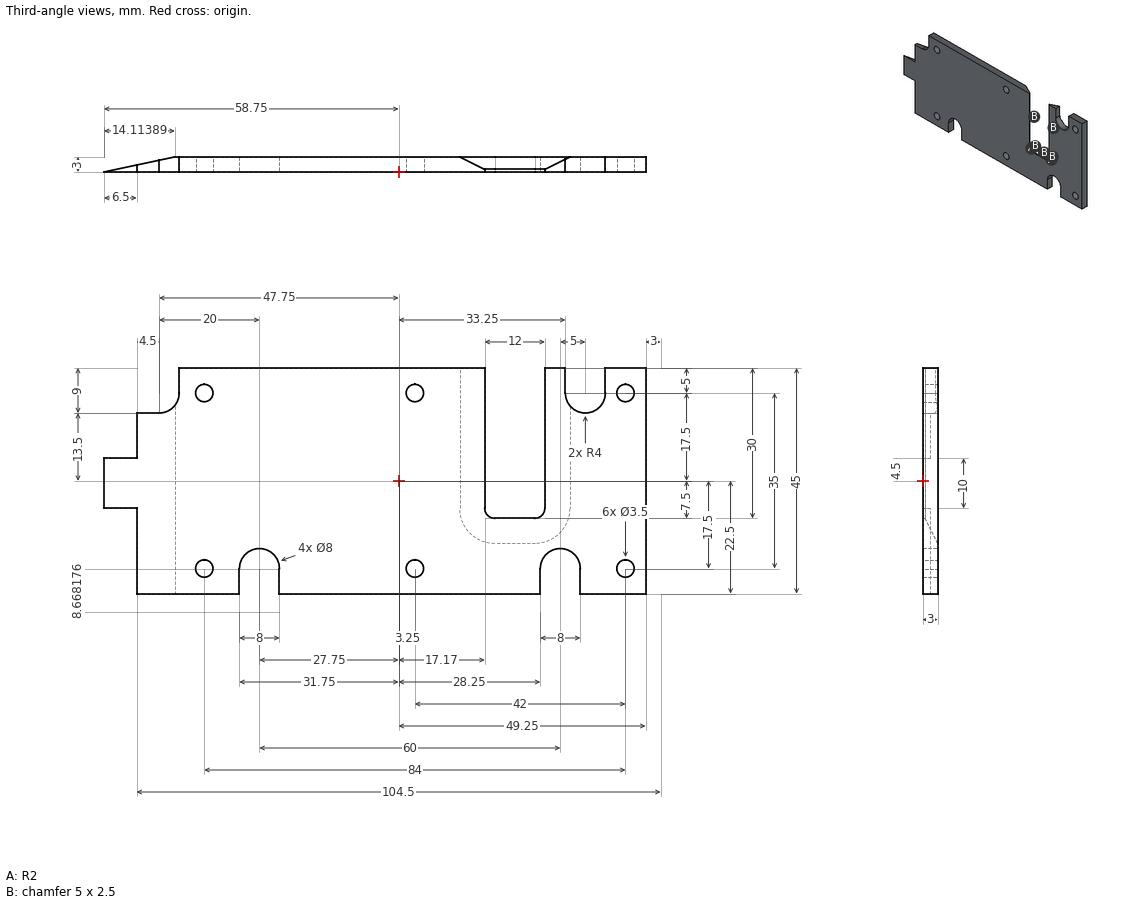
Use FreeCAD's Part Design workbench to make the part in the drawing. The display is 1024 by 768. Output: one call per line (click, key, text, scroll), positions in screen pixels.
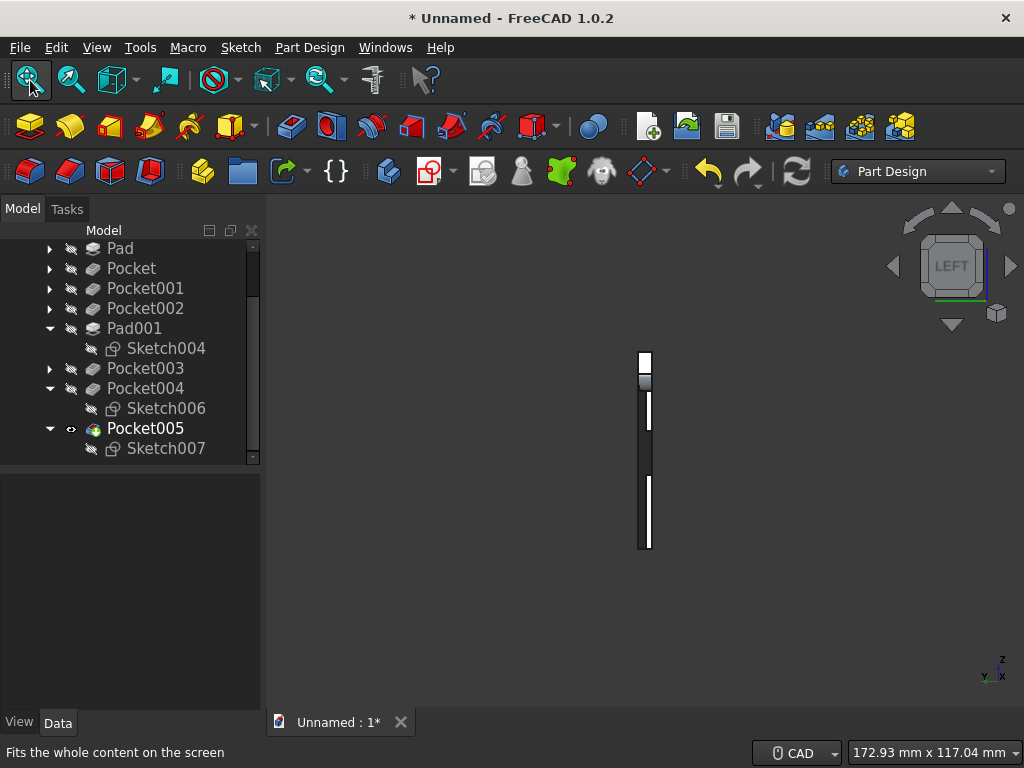
scroll(645, 482, up, 6)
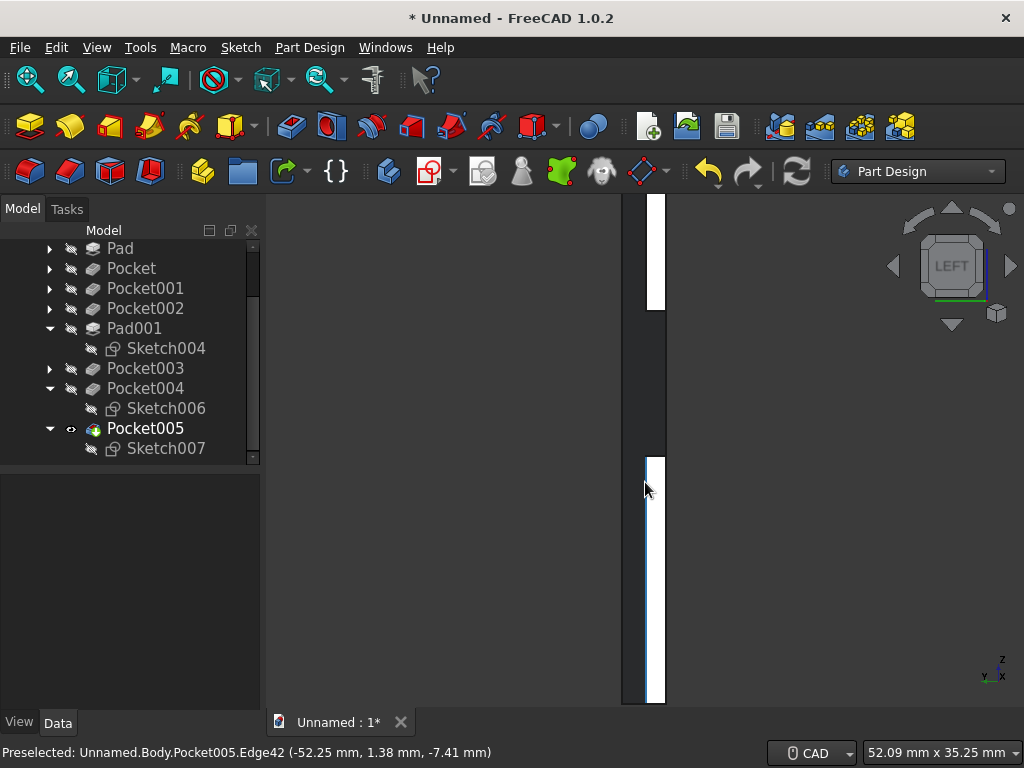
click(32, 80)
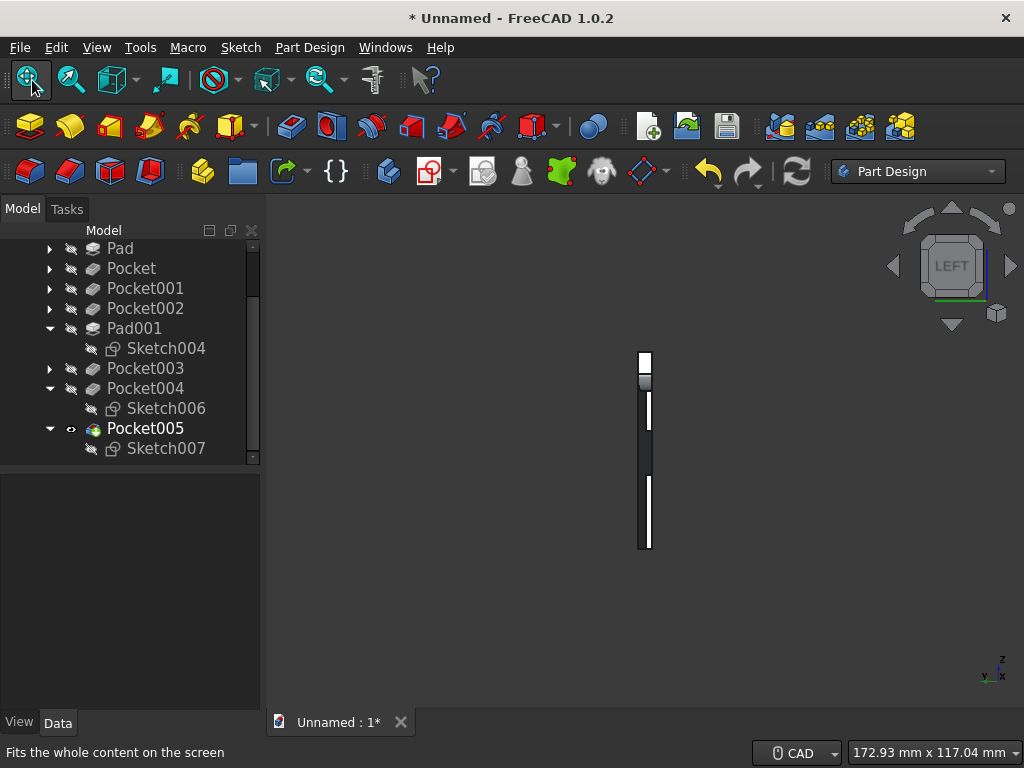
key(v)
key(3)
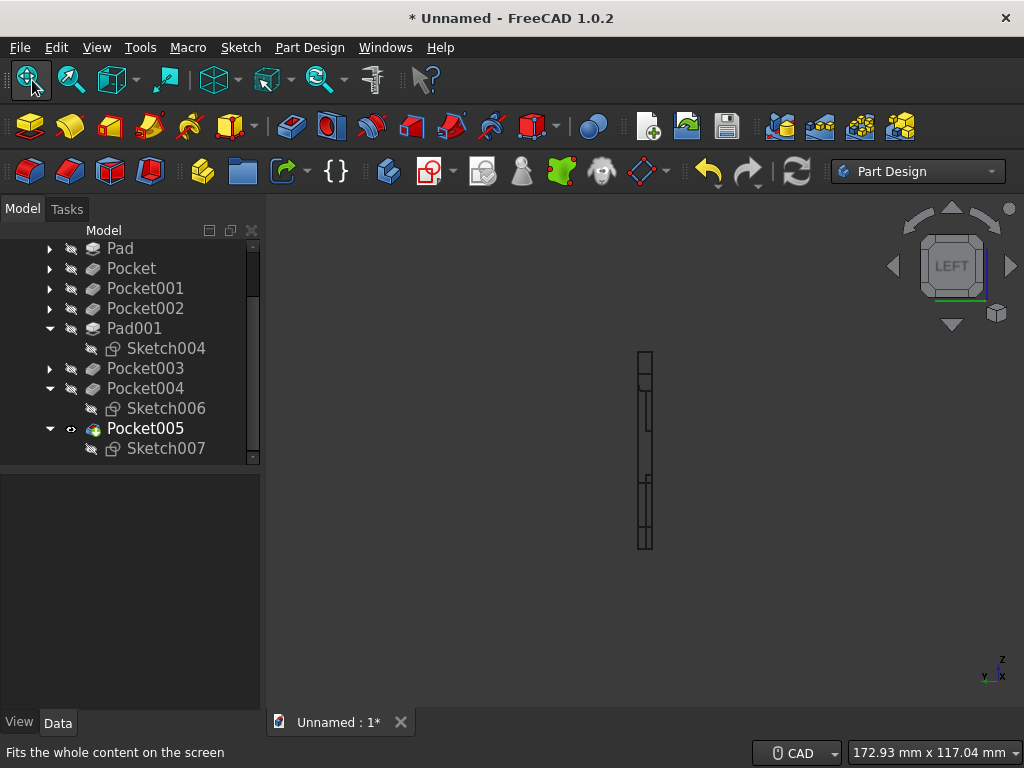
key(0)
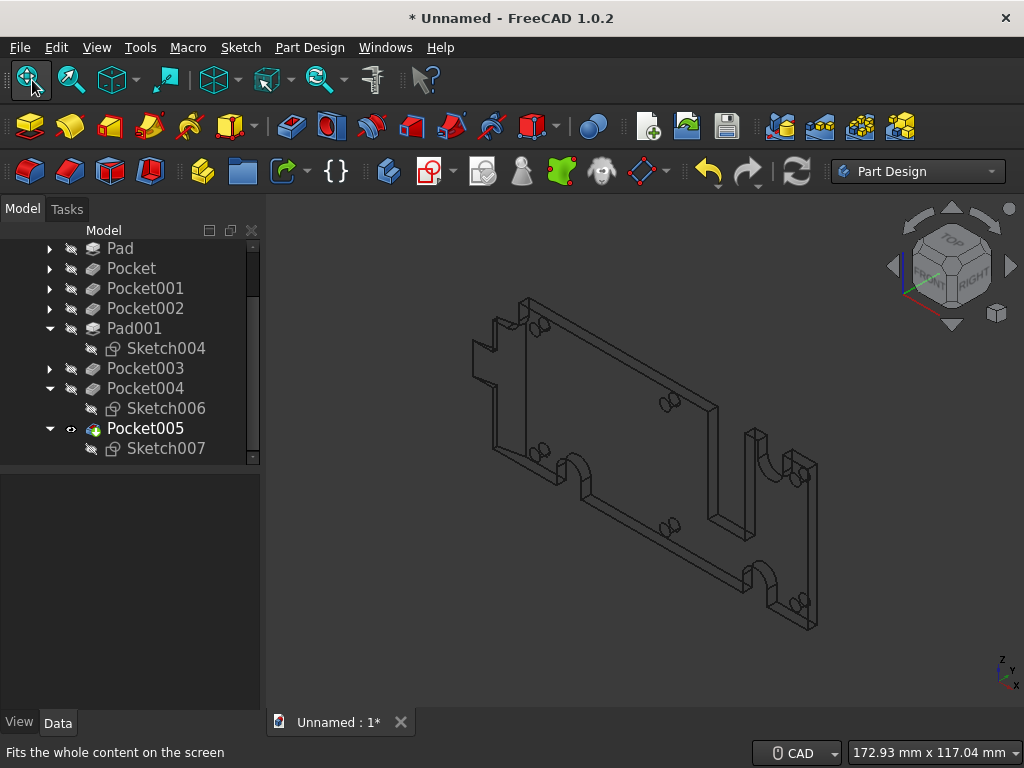
click(752, 536)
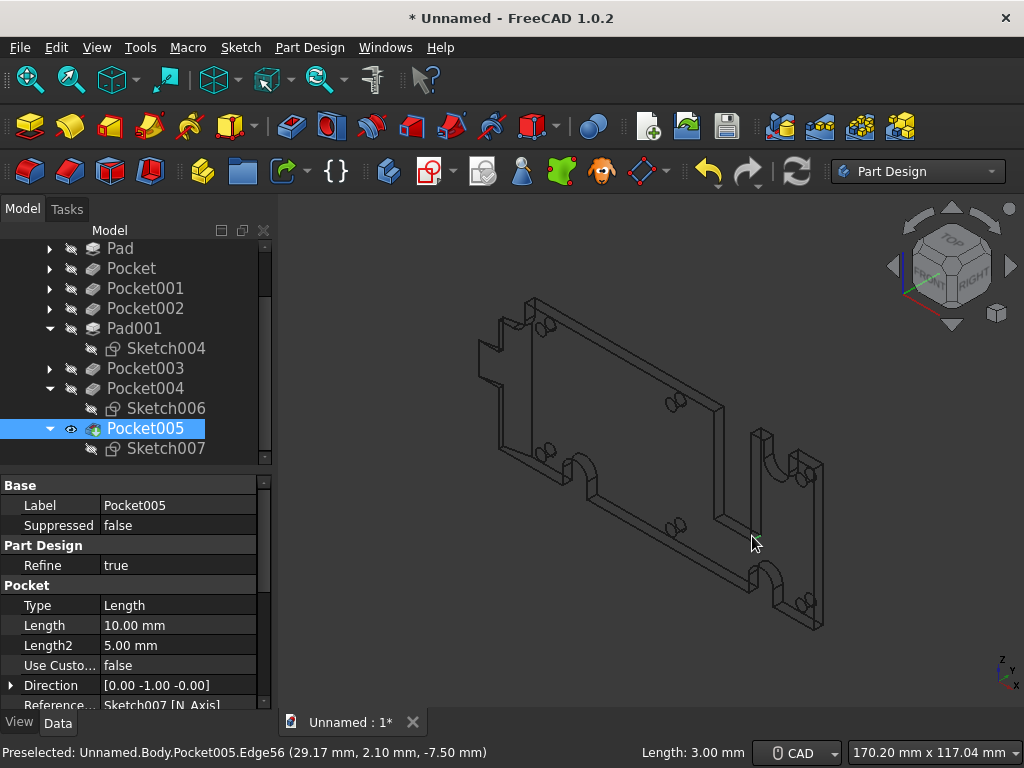
click(721, 514, ctrl)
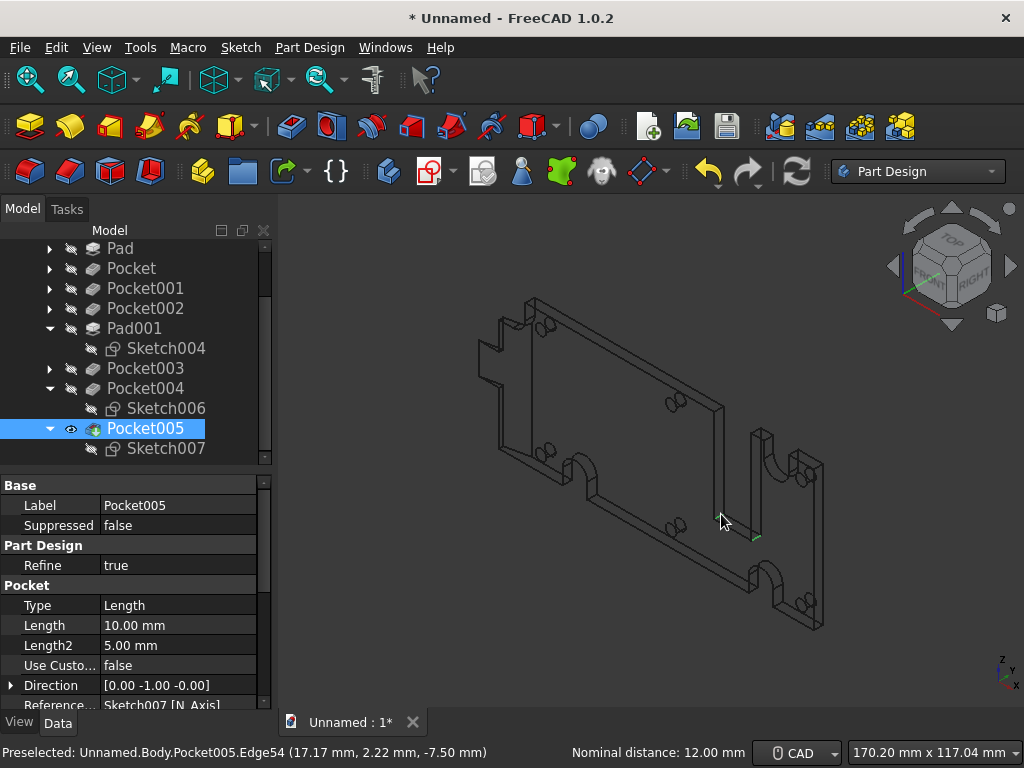
key(v)
key(1)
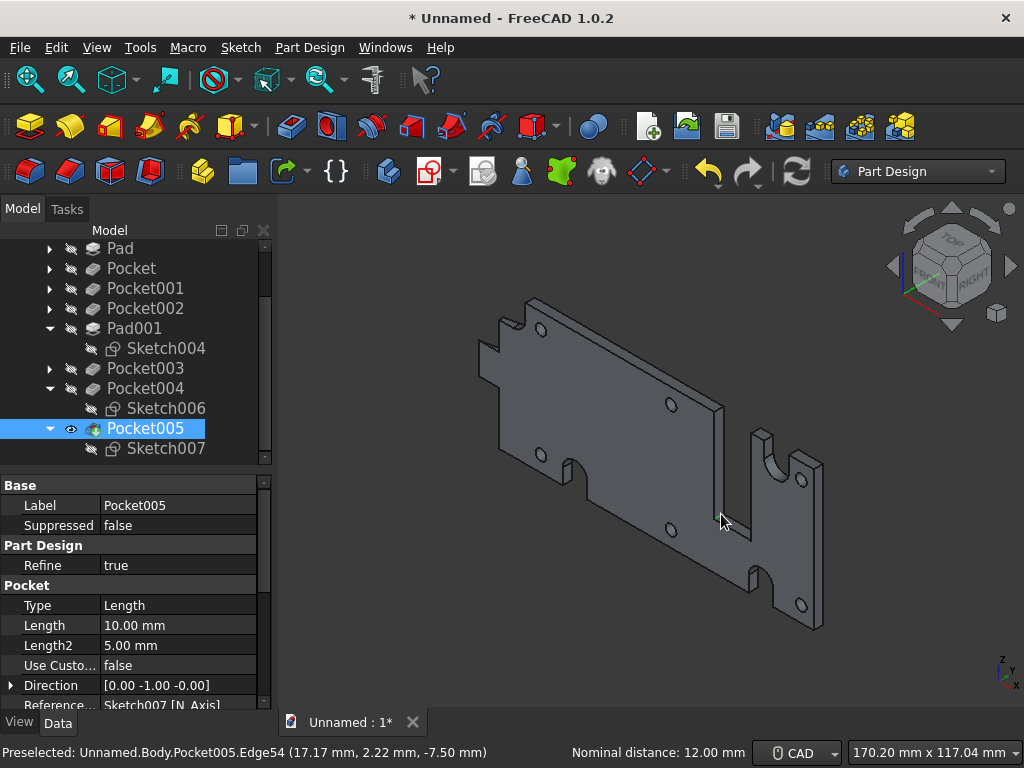
click(30, 172)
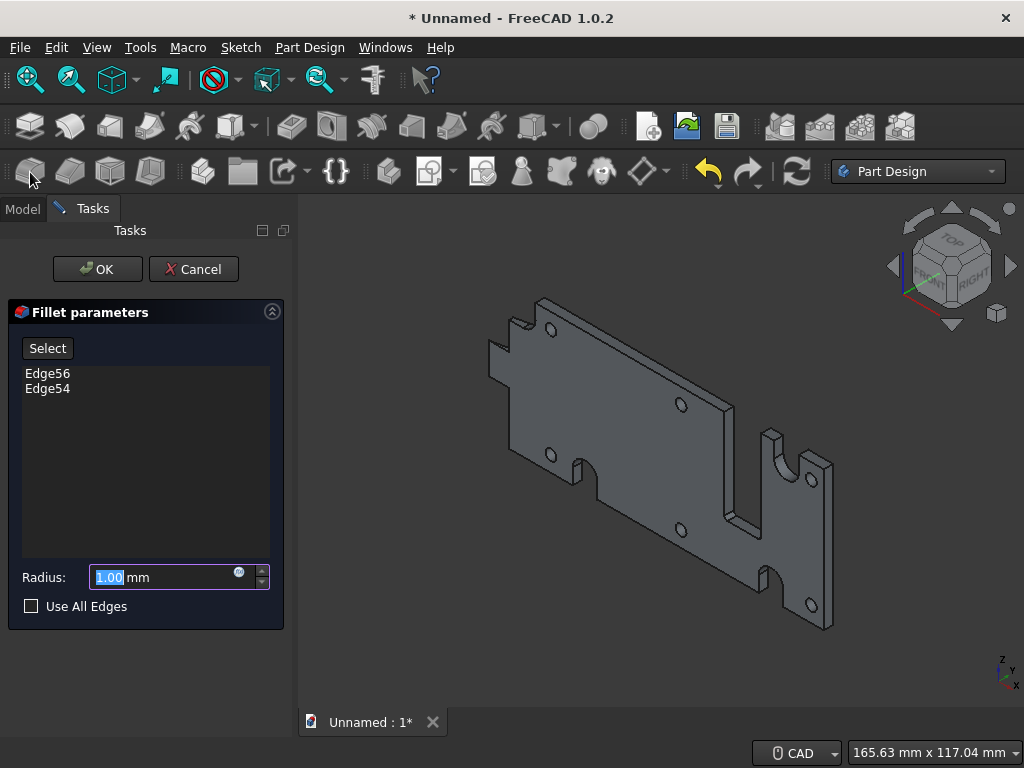
text(2)
key(Tab)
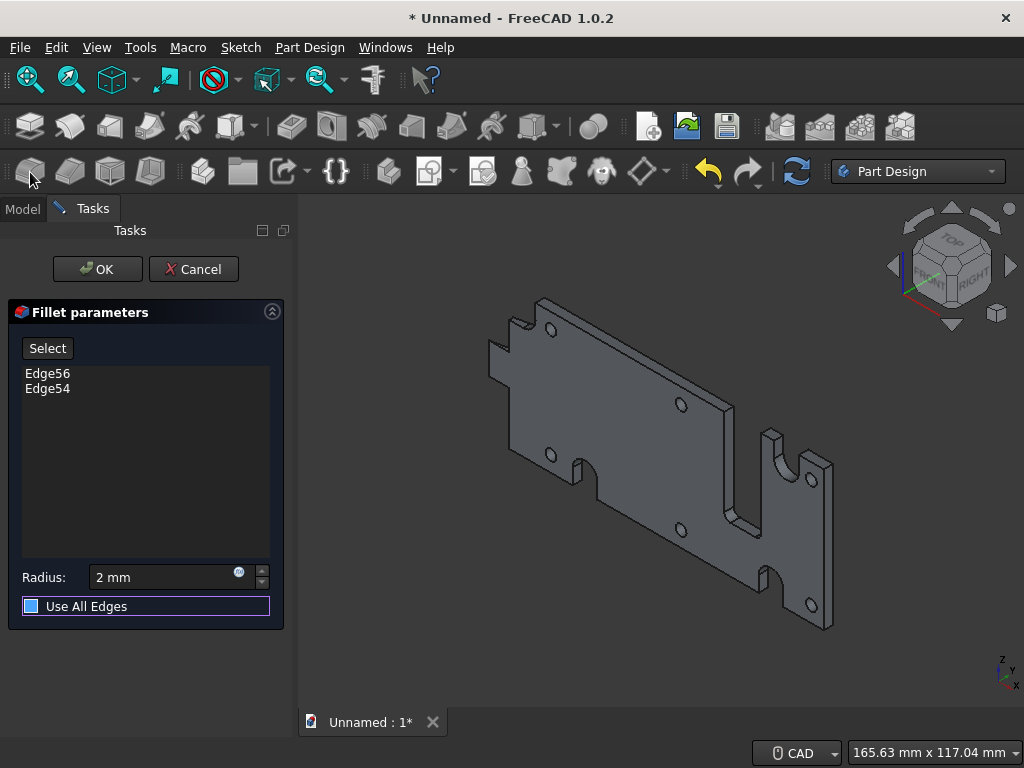
click(98, 269)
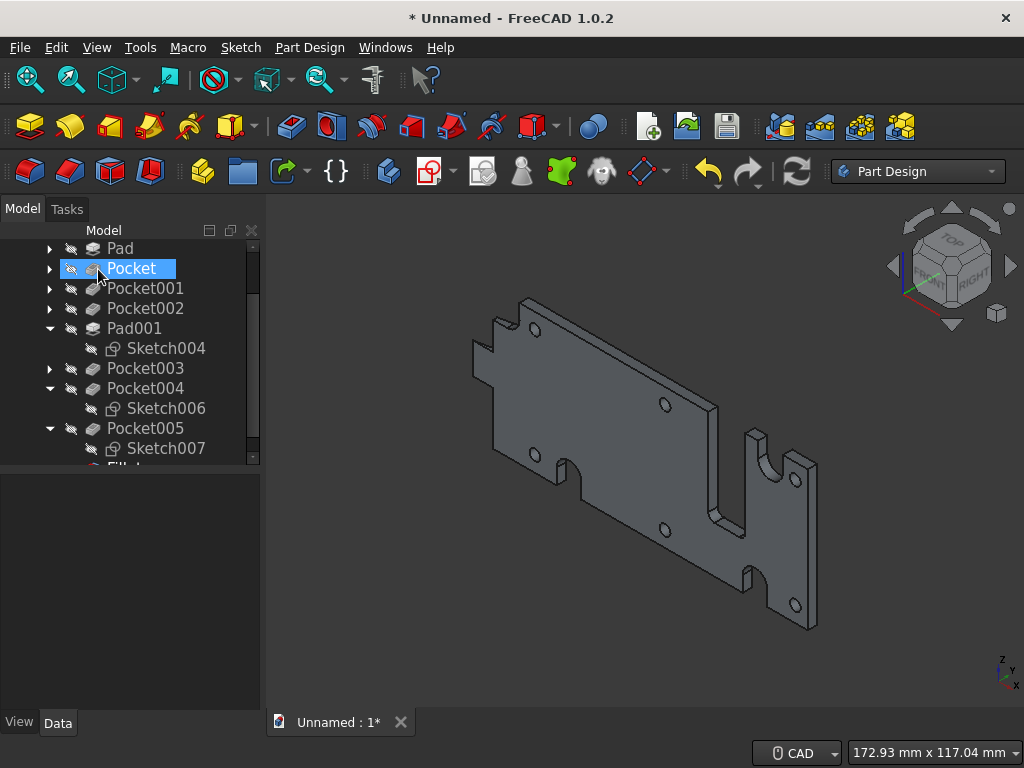
key(2)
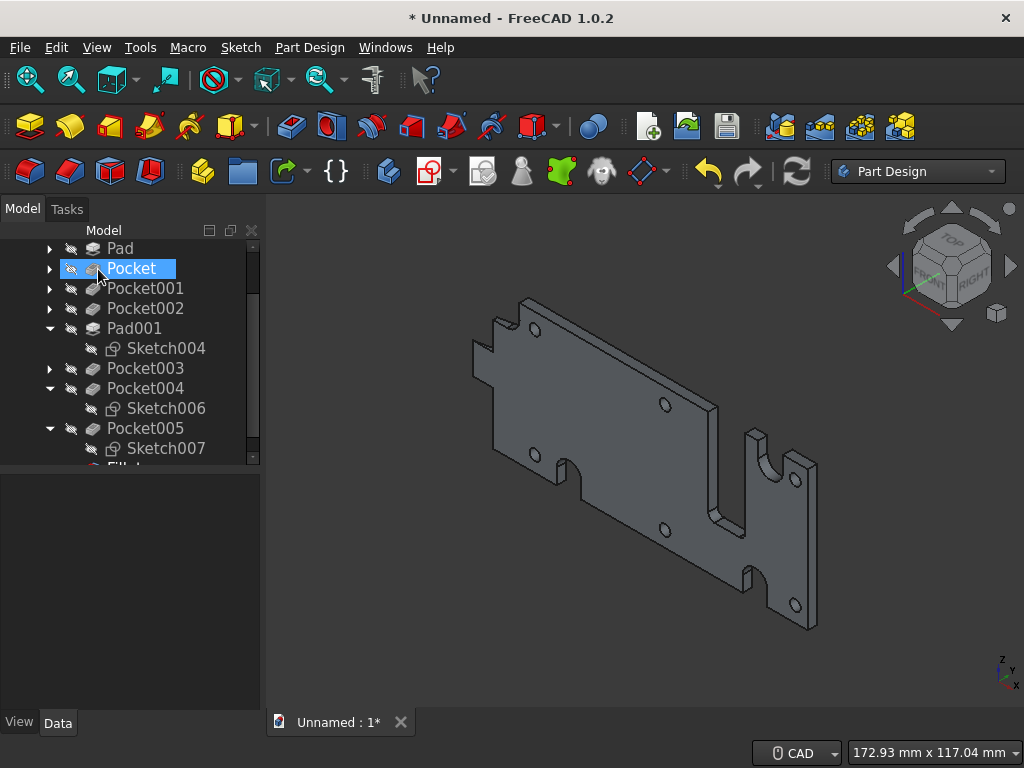
click(787, 443)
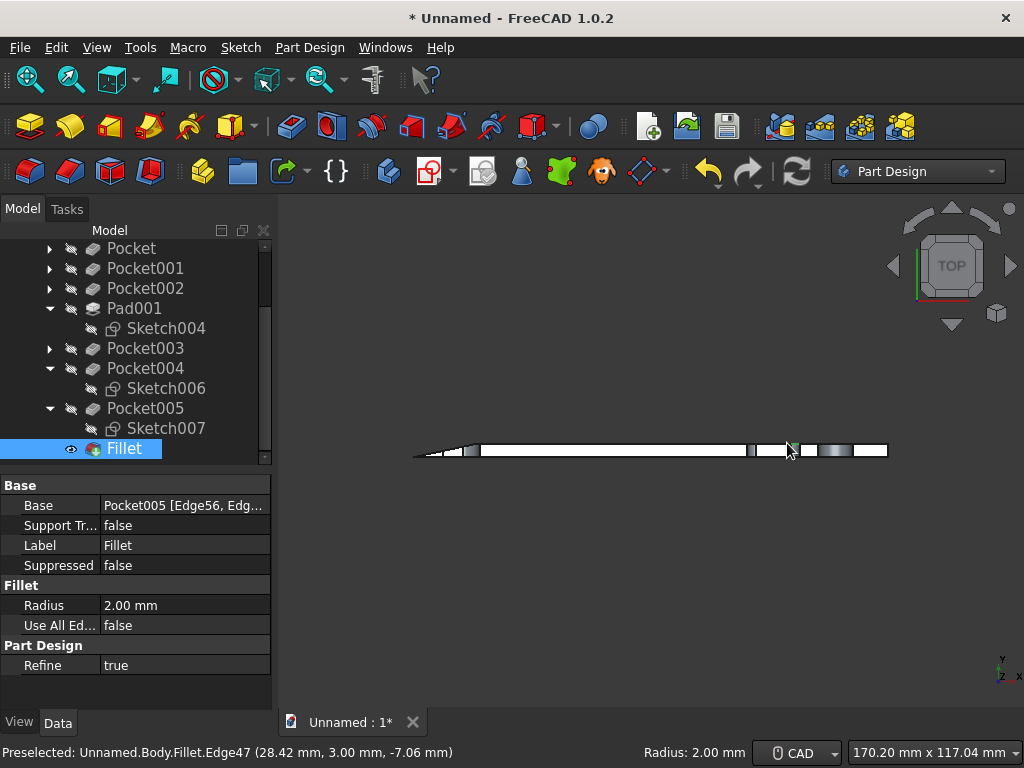
click(773, 443, ctrl)